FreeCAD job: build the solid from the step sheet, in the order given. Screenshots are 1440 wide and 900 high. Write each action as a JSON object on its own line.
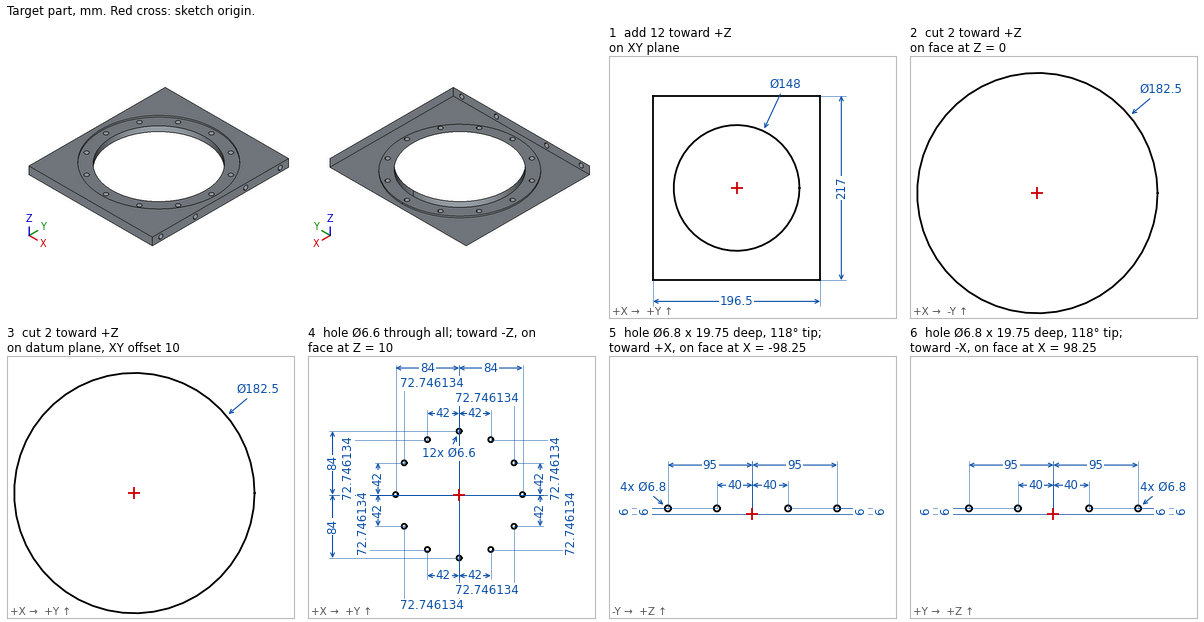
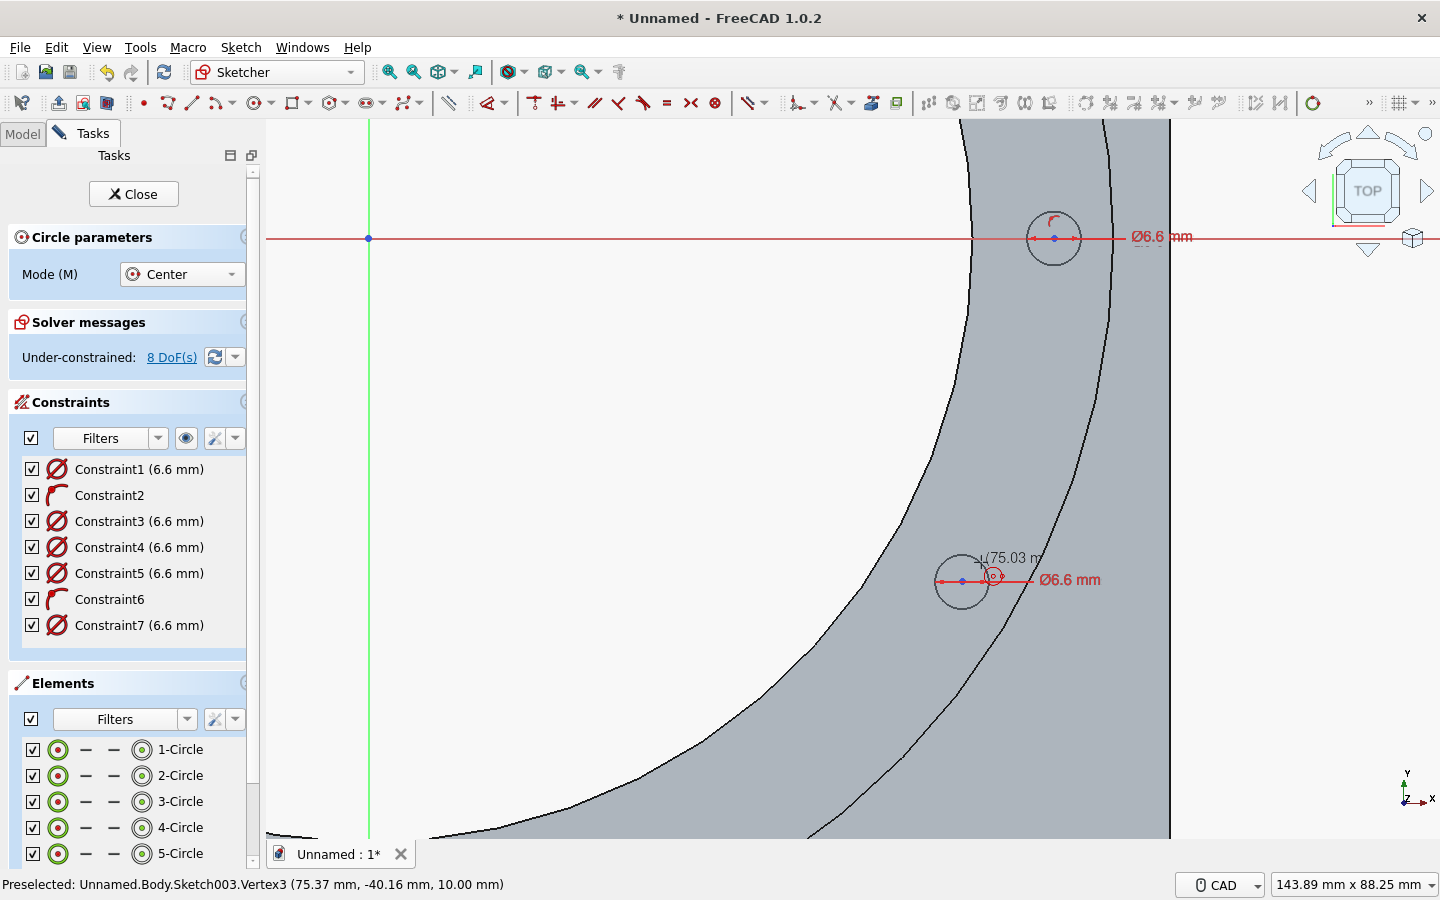
{"action": "scroll", "coordinate": [964, 583], "scroll_direction": "down", "scroll_amount": 6}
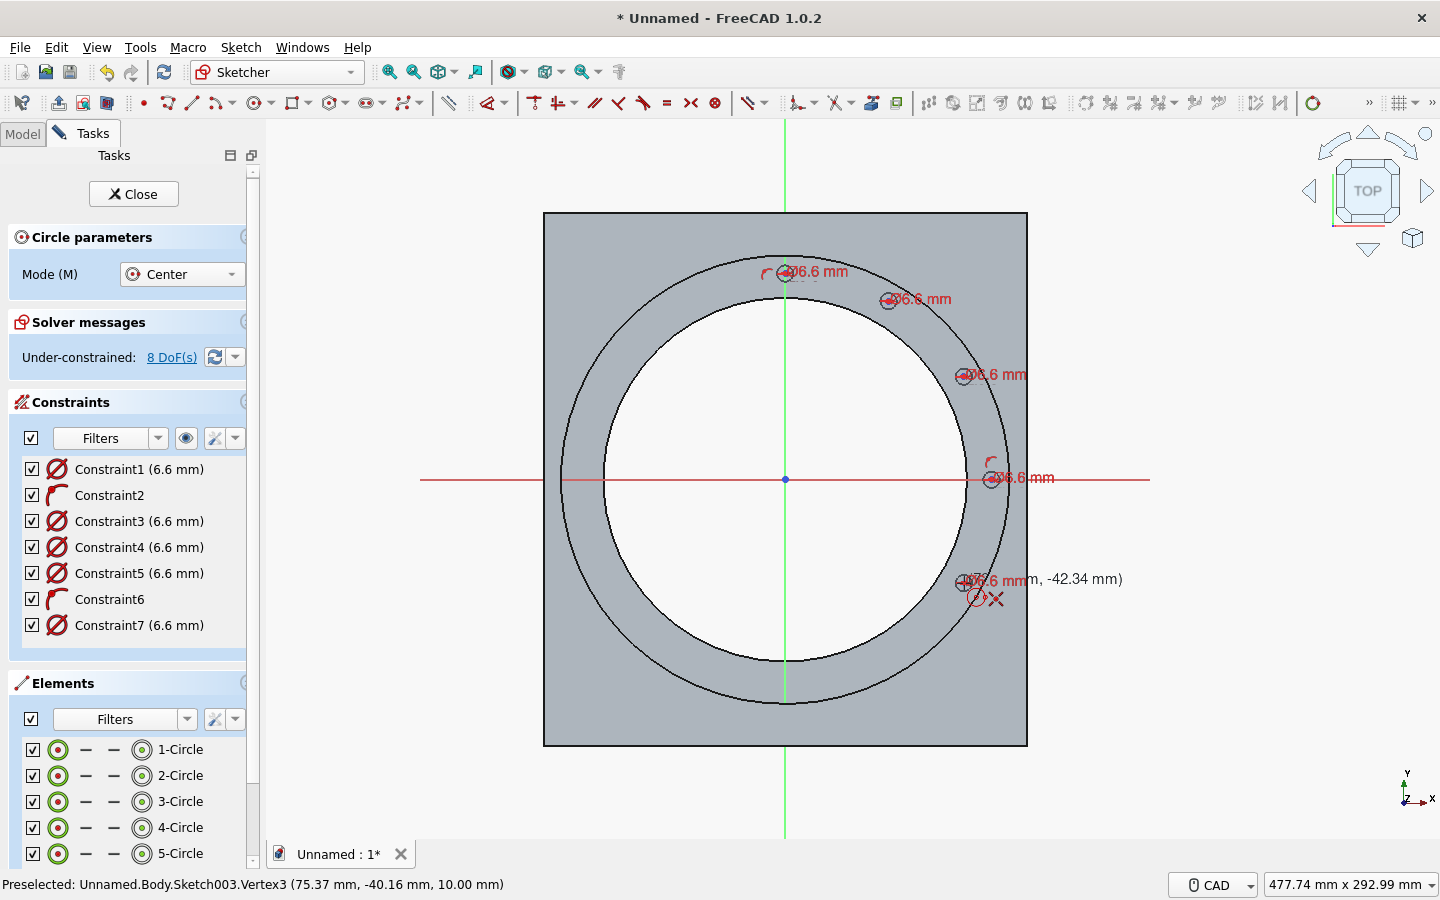
{"action": "scroll", "coordinate": [888, 658], "scroll_direction": "up", "scroll_amount": 6}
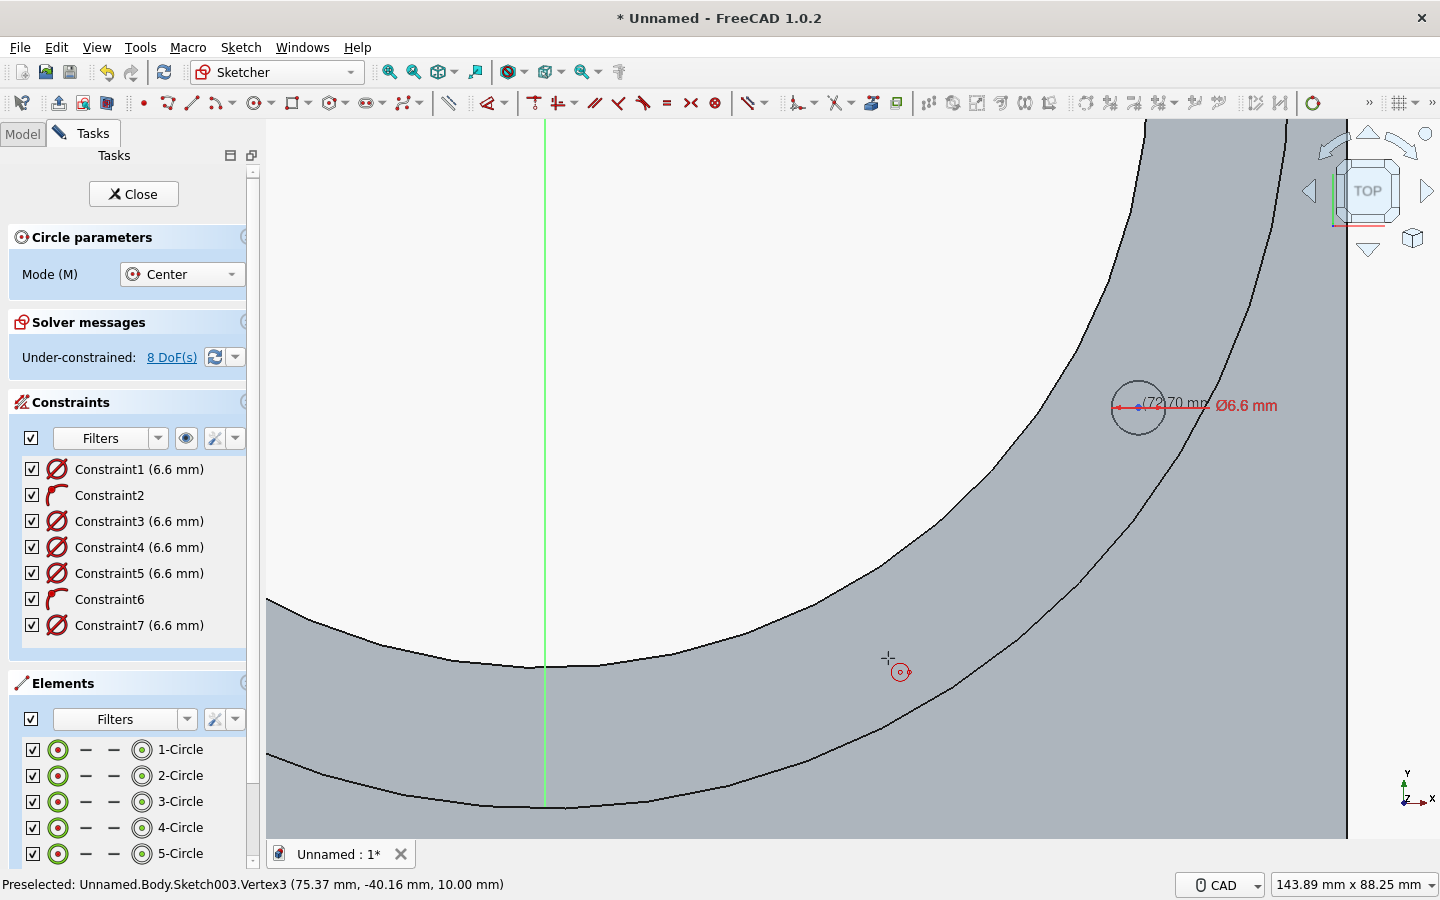
{"action": "left_click", "coordinate": [888, 658]}
{"action": "mouse_move", "coordinate": [907, 639]}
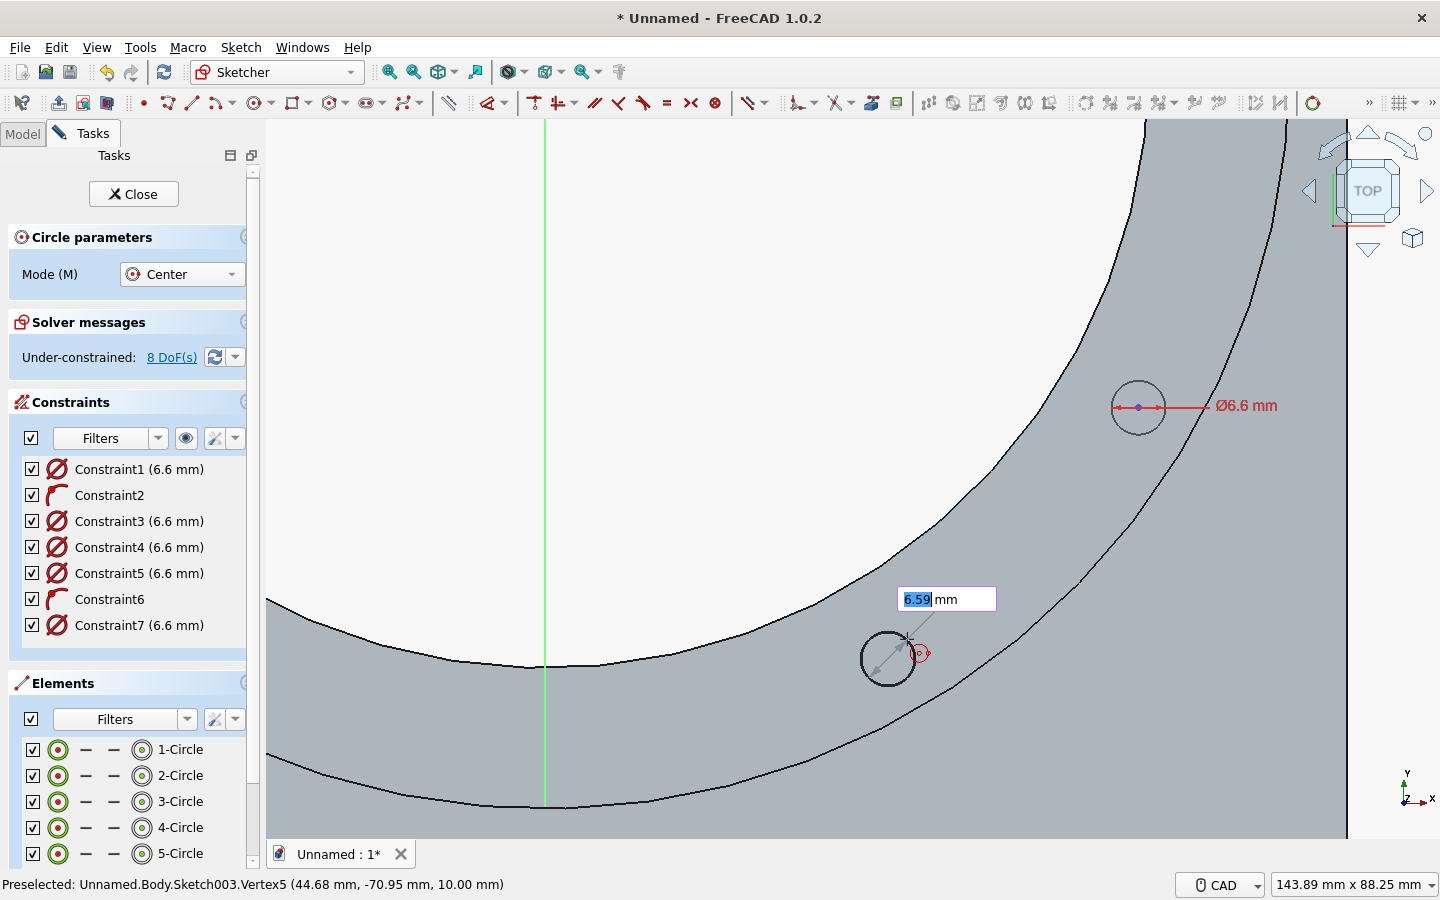
{"action": "type", "text": "6.6"}
{"action": "key", "text": "Return"}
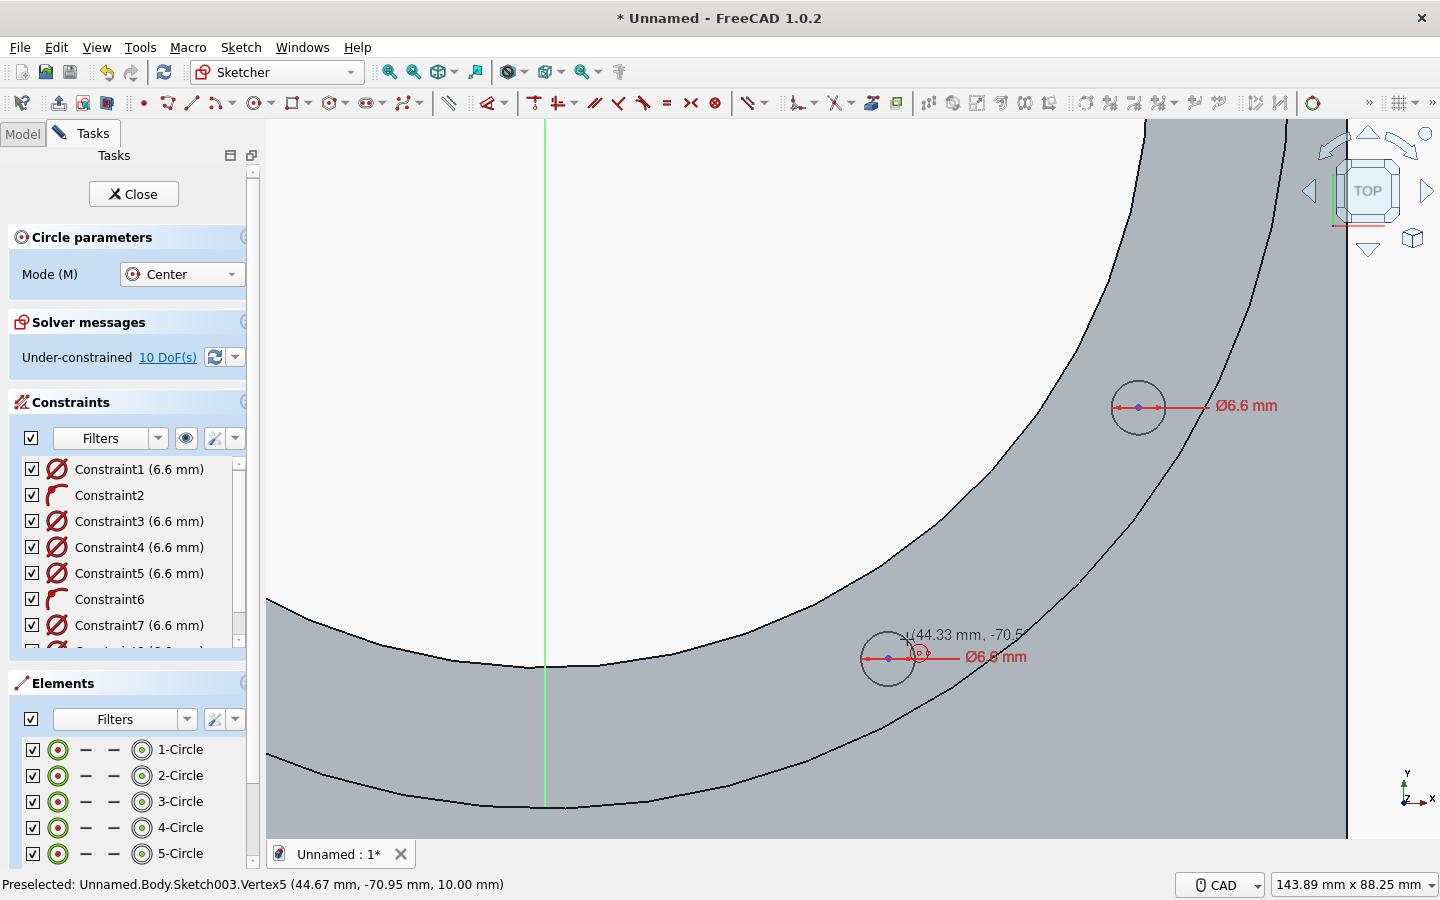
{"action": "left_click", "coordinate": [545, 750]}
{"action": "mouse_move", "coordinate": [564, 731]}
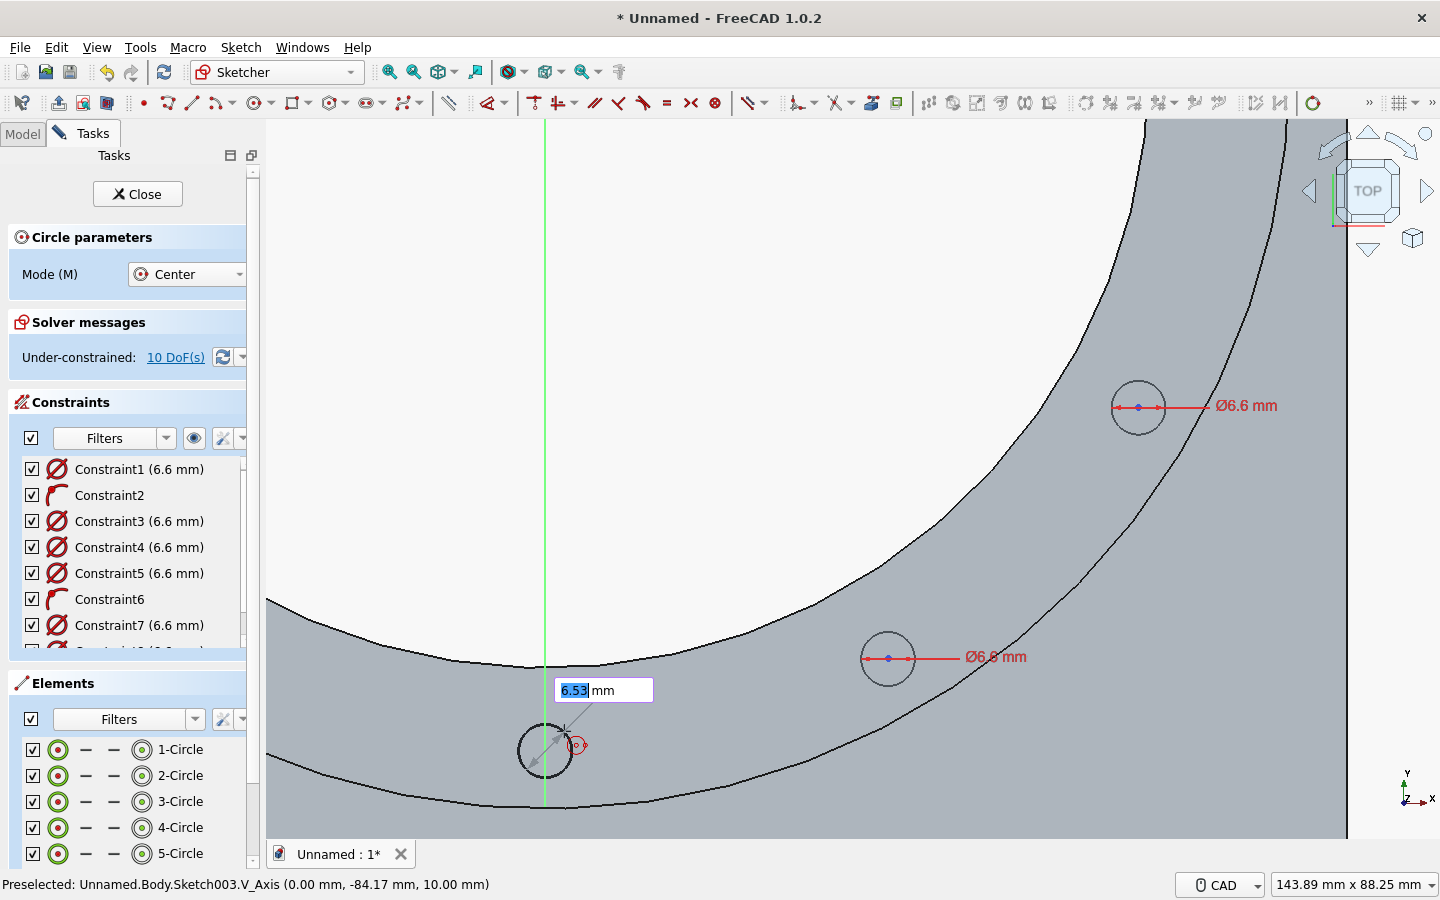
{"action": "type", "text": "6.6"}
{"action": "key", "text": "Return"}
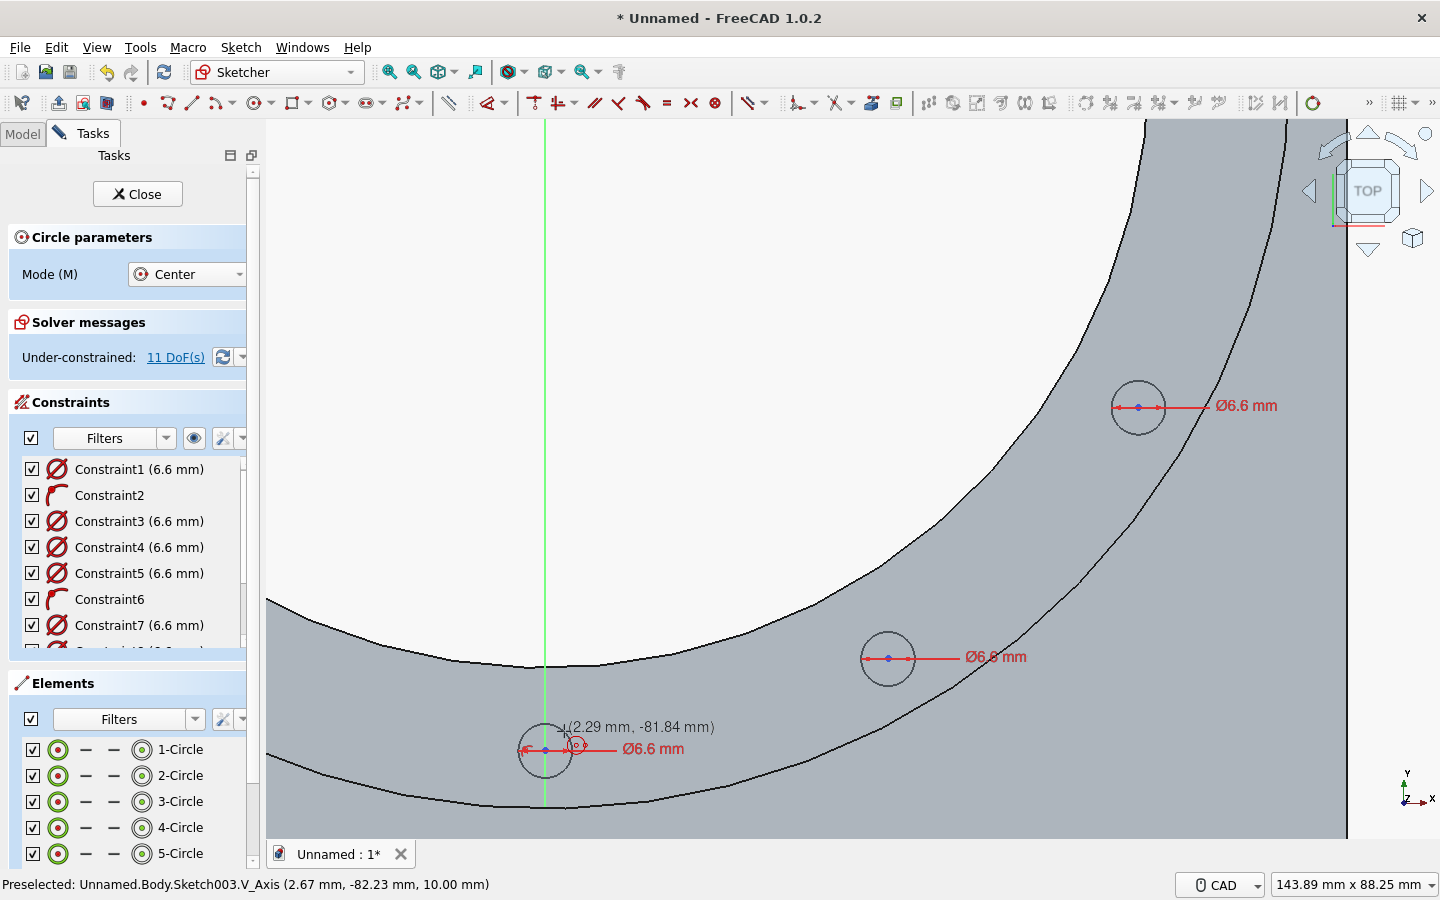
{"action": "scroll", "coordinate": [888, 658], "scroll_direction": "down", "scroll_amount": 6}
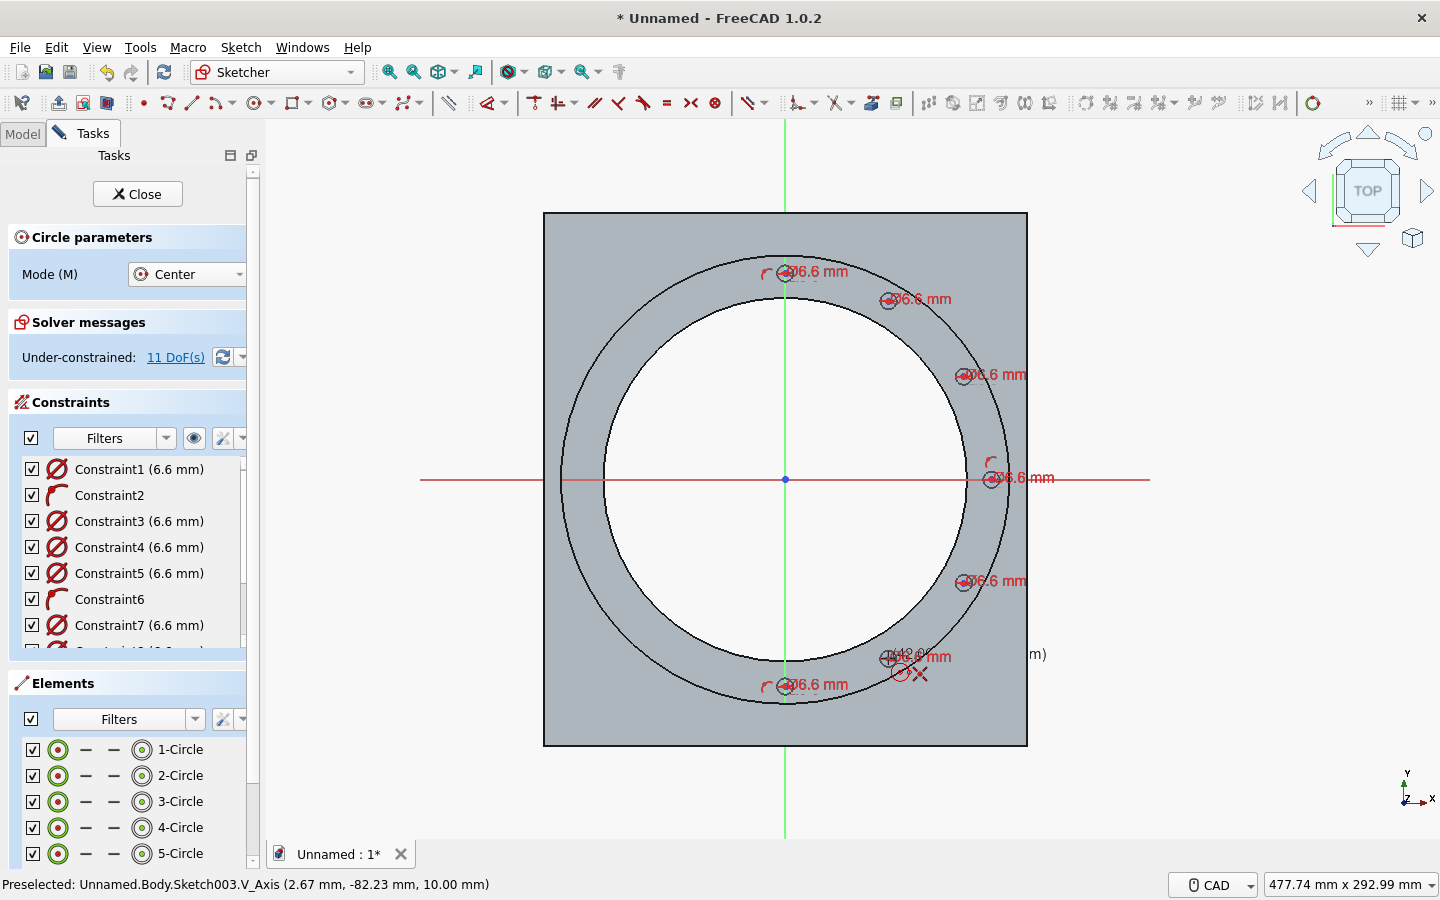
{"action": "scroll", "coordinate": [682, 658], "scroll_direction": "up", "scroll_amount": 6}